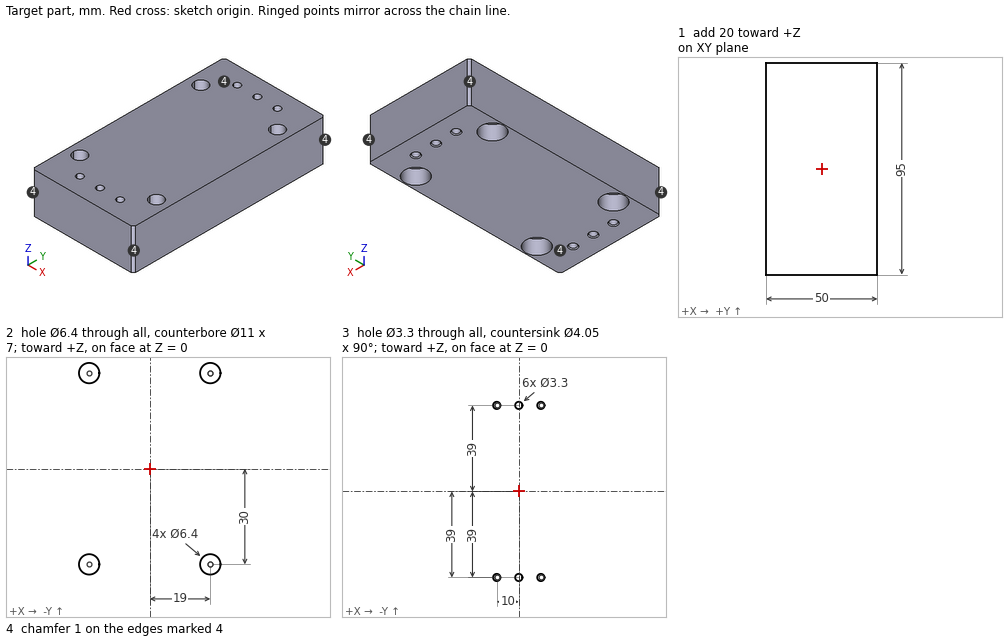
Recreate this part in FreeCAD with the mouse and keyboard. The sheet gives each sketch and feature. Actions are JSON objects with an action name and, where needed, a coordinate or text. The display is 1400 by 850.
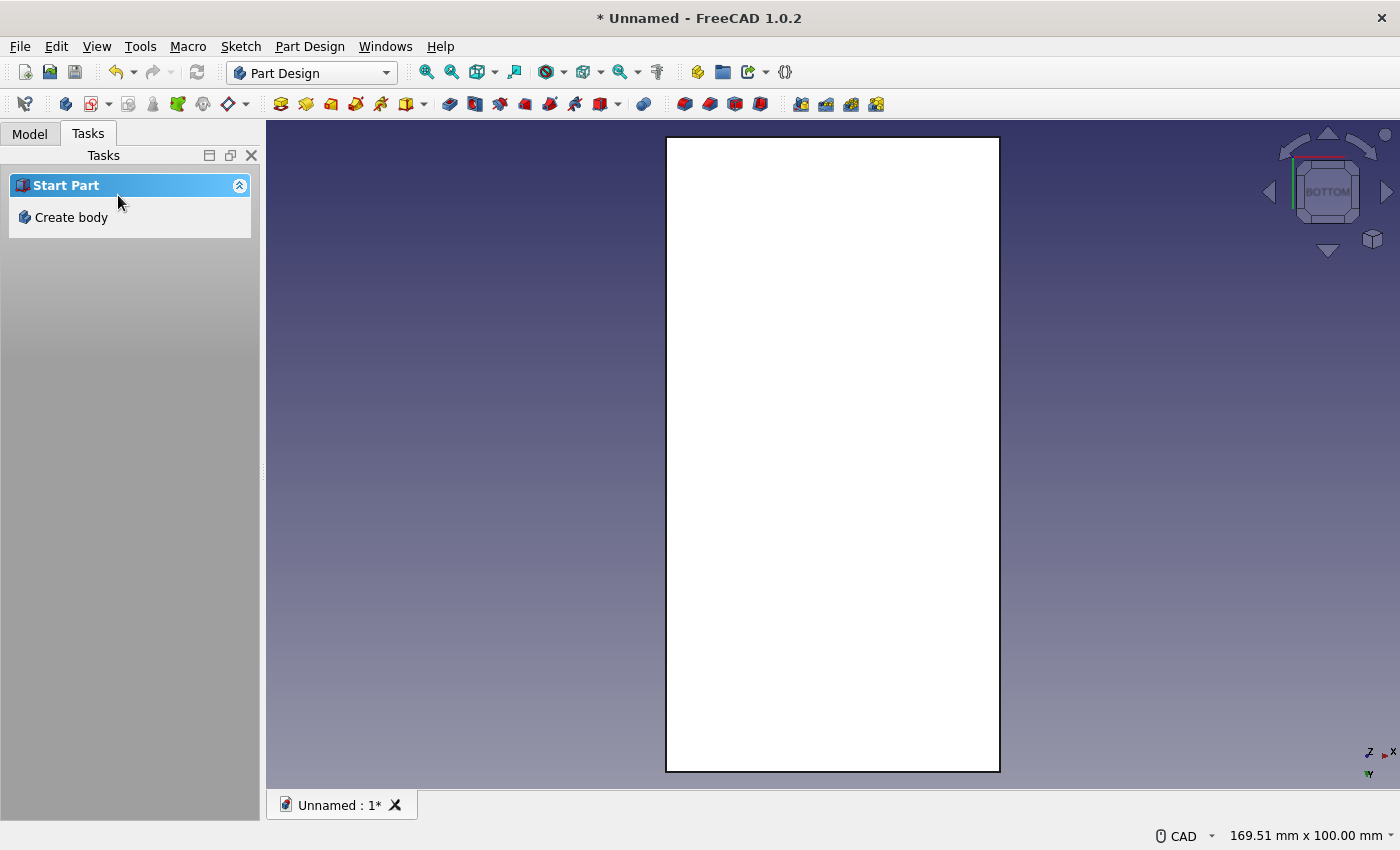
{"action": "left_click", "coordinate": [833, 544]}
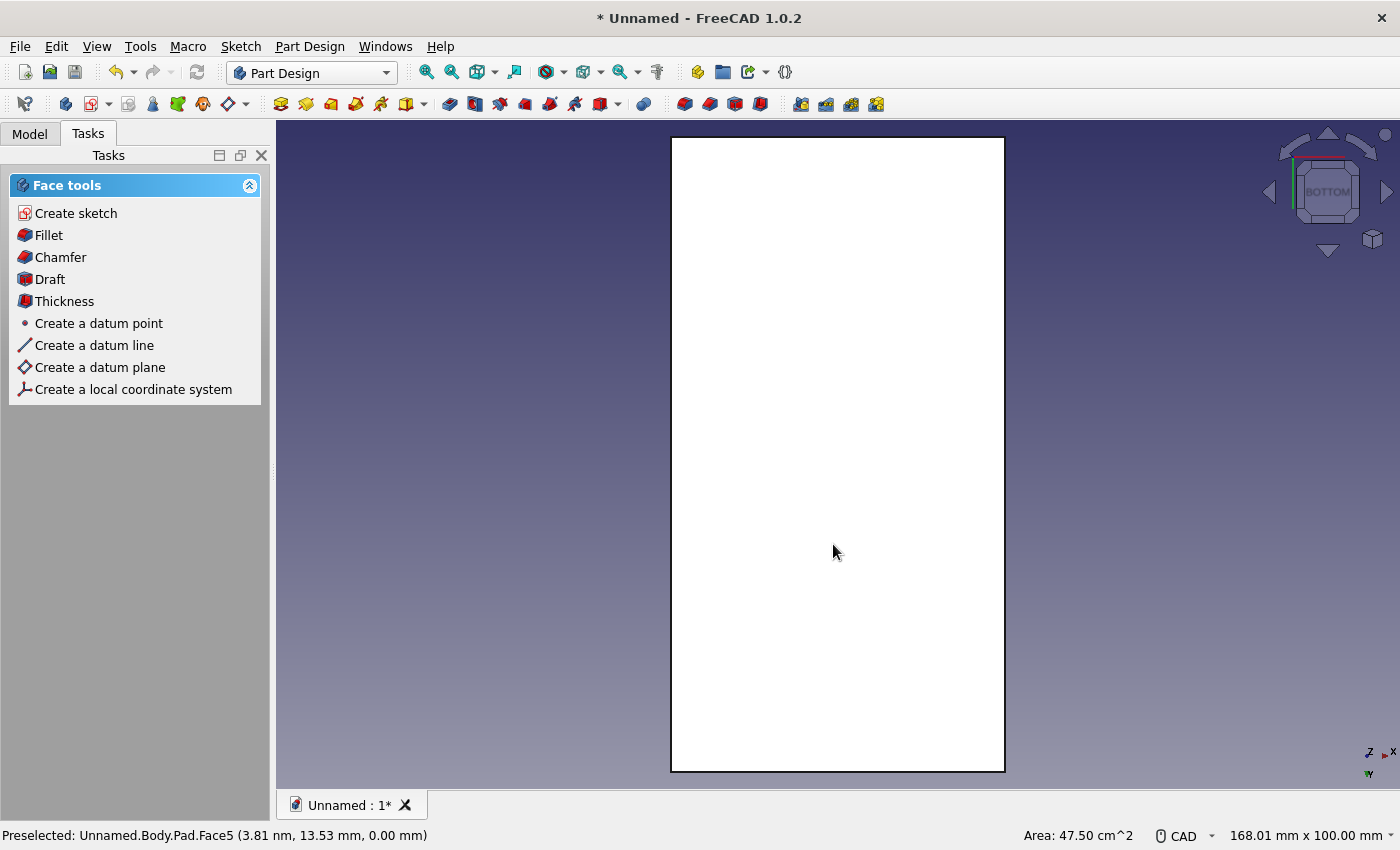
{"action": "left_click", "coordinate": [90, 104]}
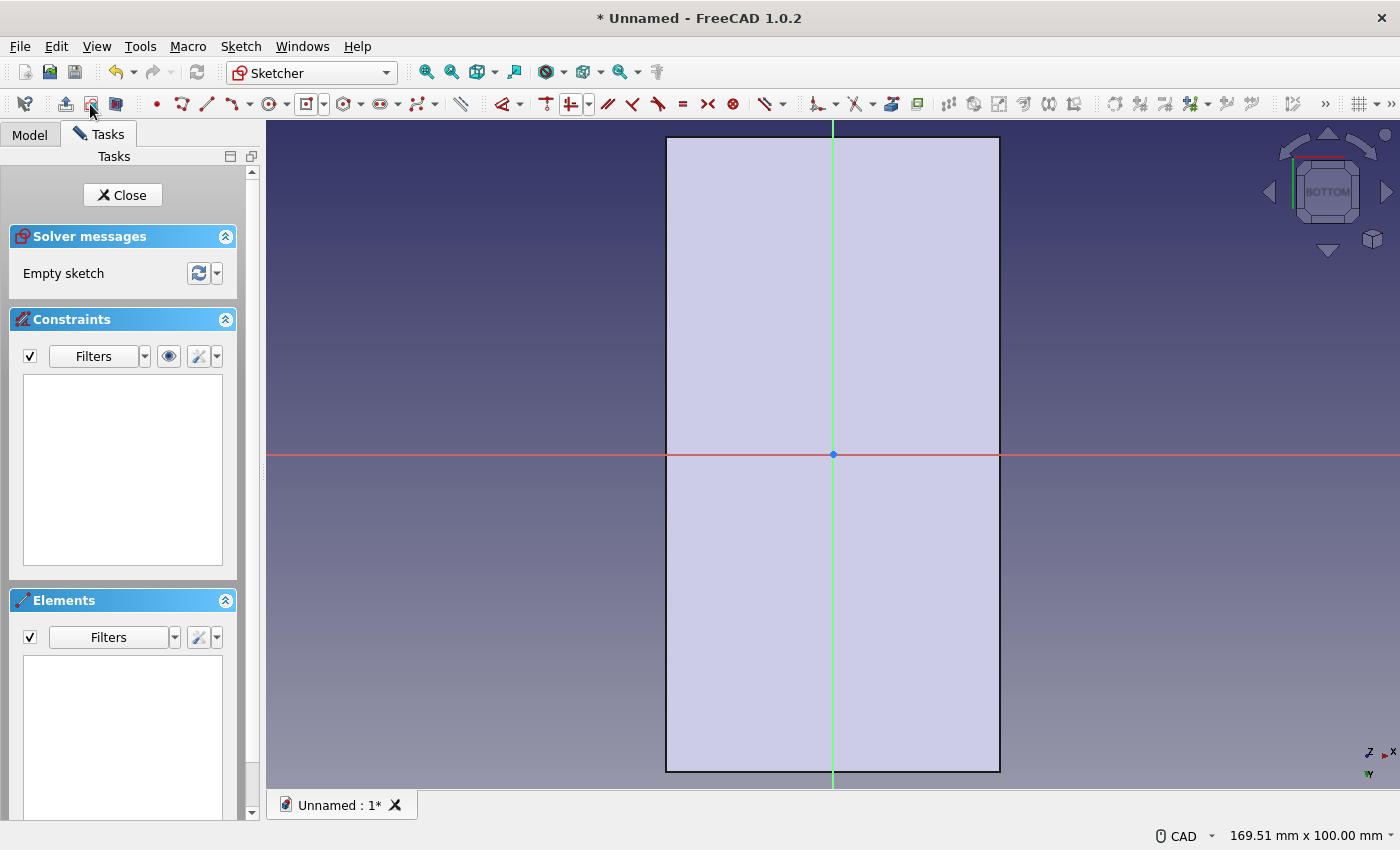
{"action": "left_click", "coordinate": [268, 104]}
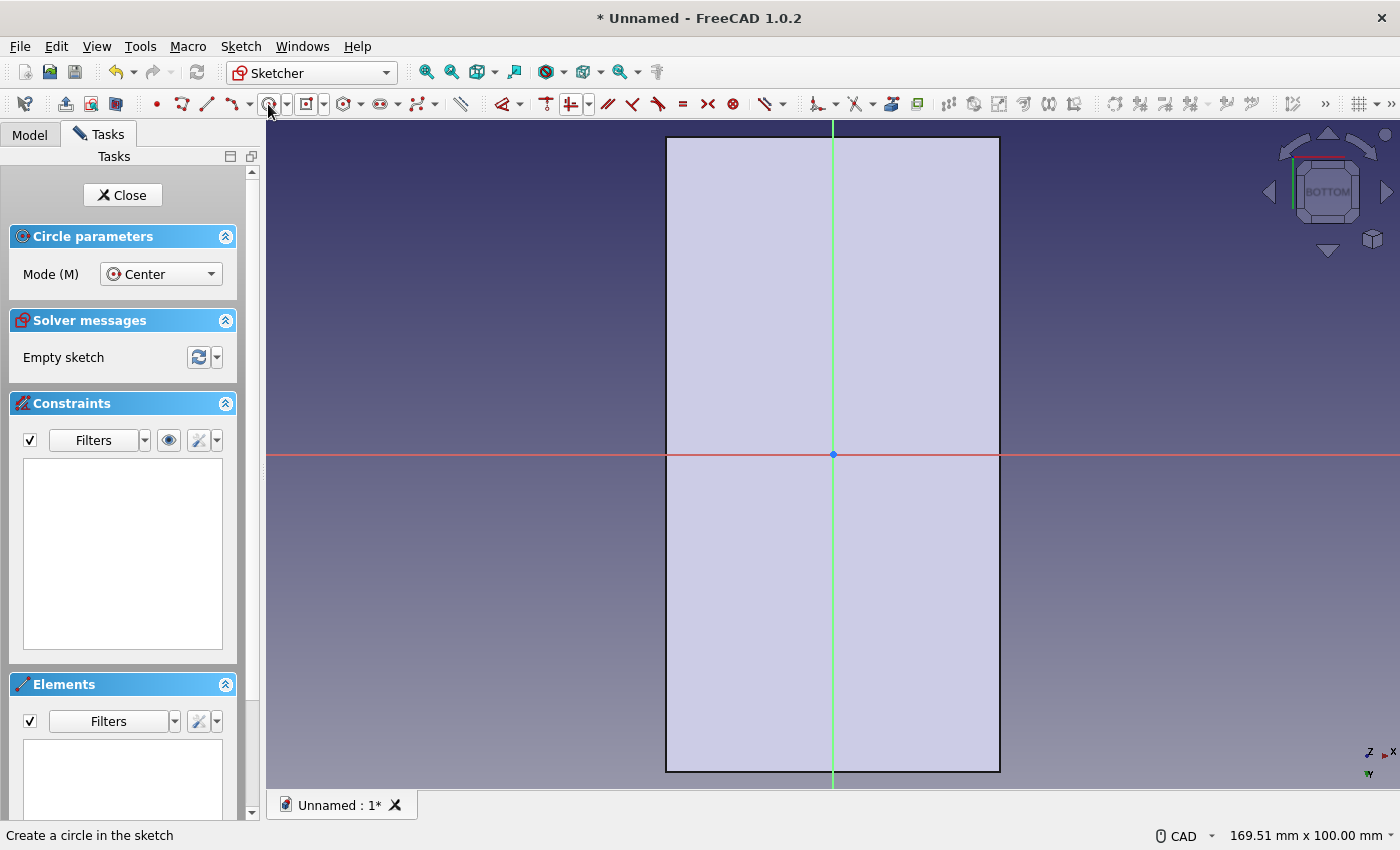
{"action": "left_click", "coordinate": [960, 655]}
{"action": "left_click", "coordinate": [975, 640]}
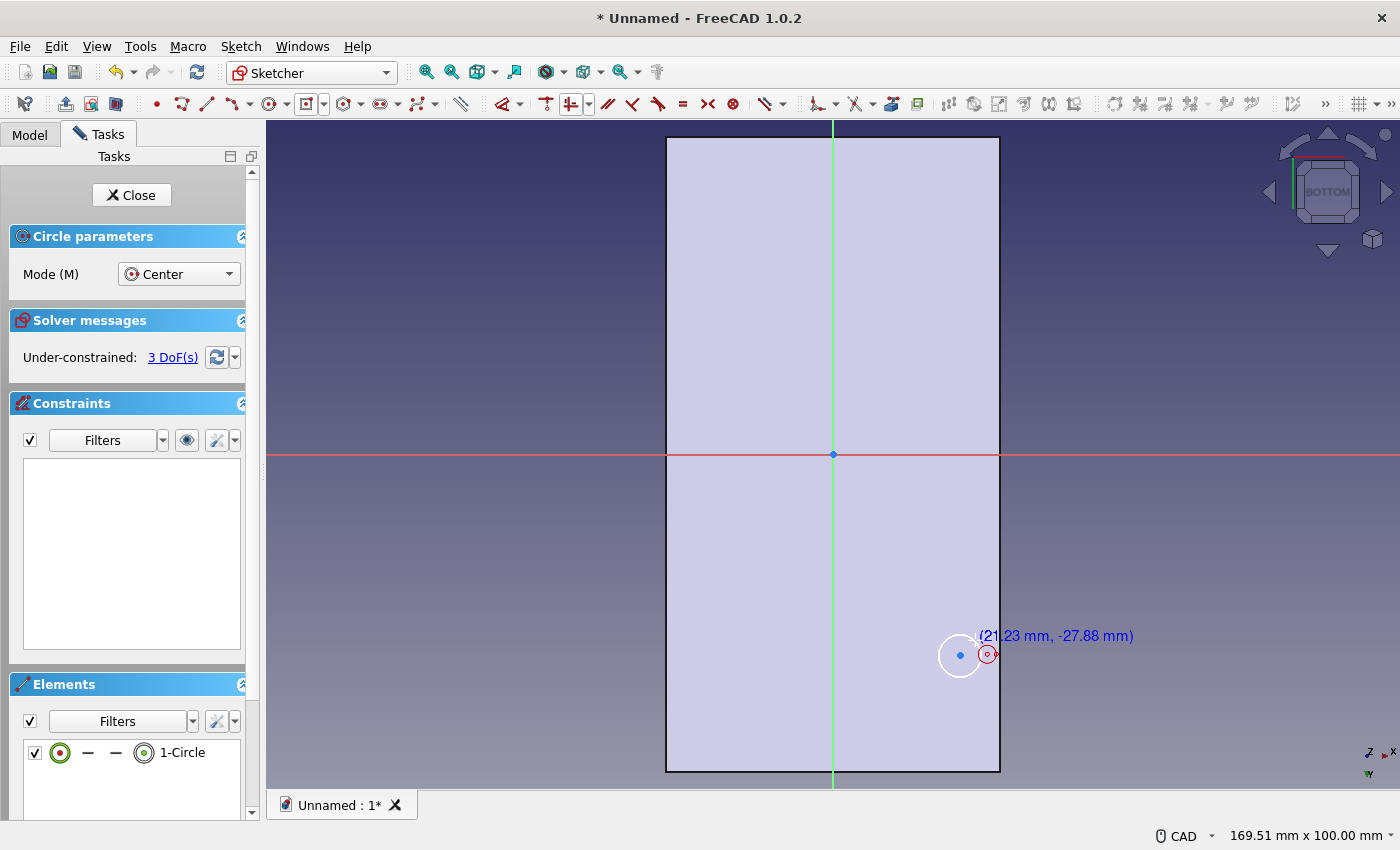
{"action": "left_click", "coordinate": [960, 254]}
{"action": "left_click", "coordinate": [975, 239]}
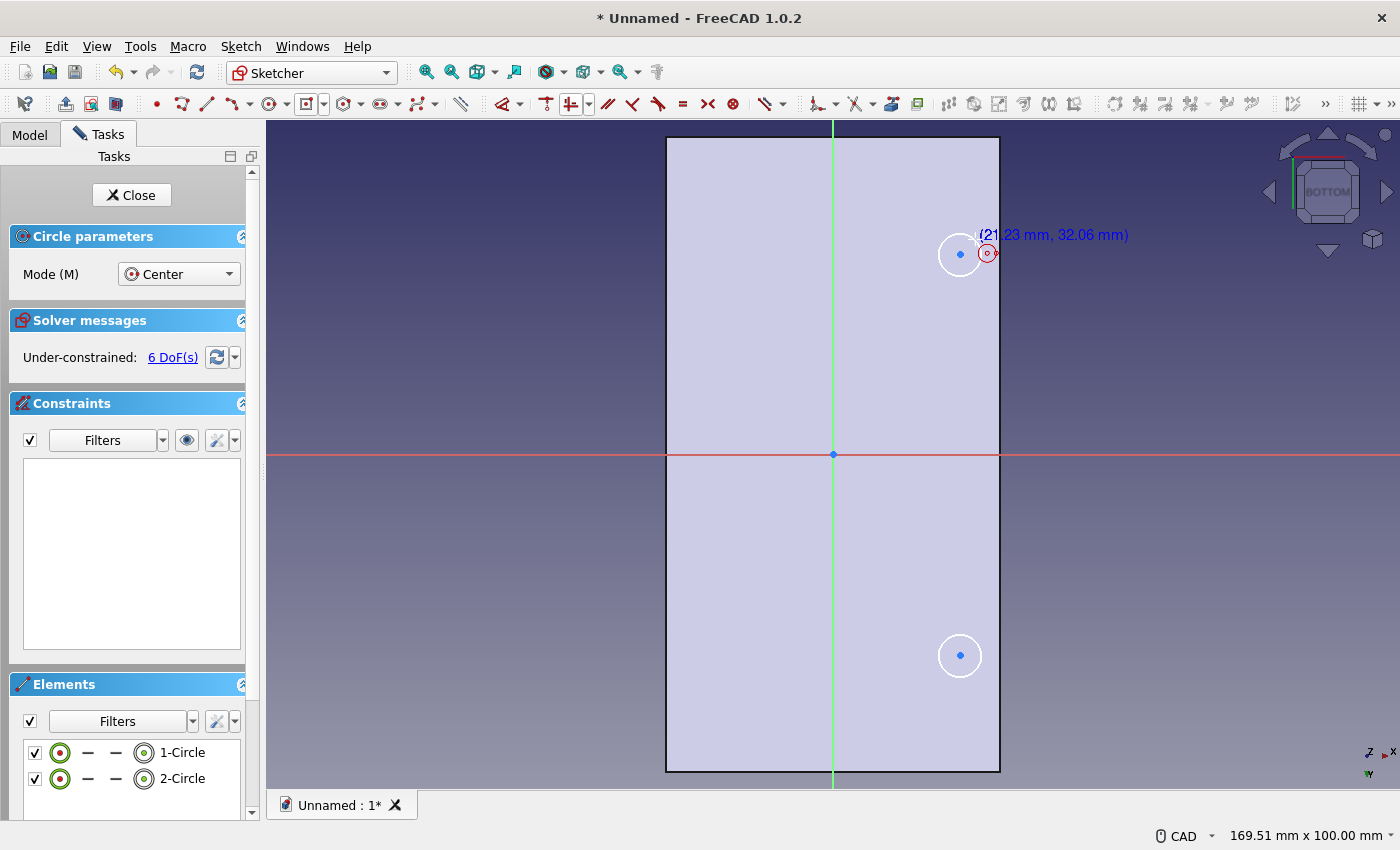
{"action": "left_click", "coordinate": [706, 254]}
{"action": "left_click", "coordinate": [721, 239]}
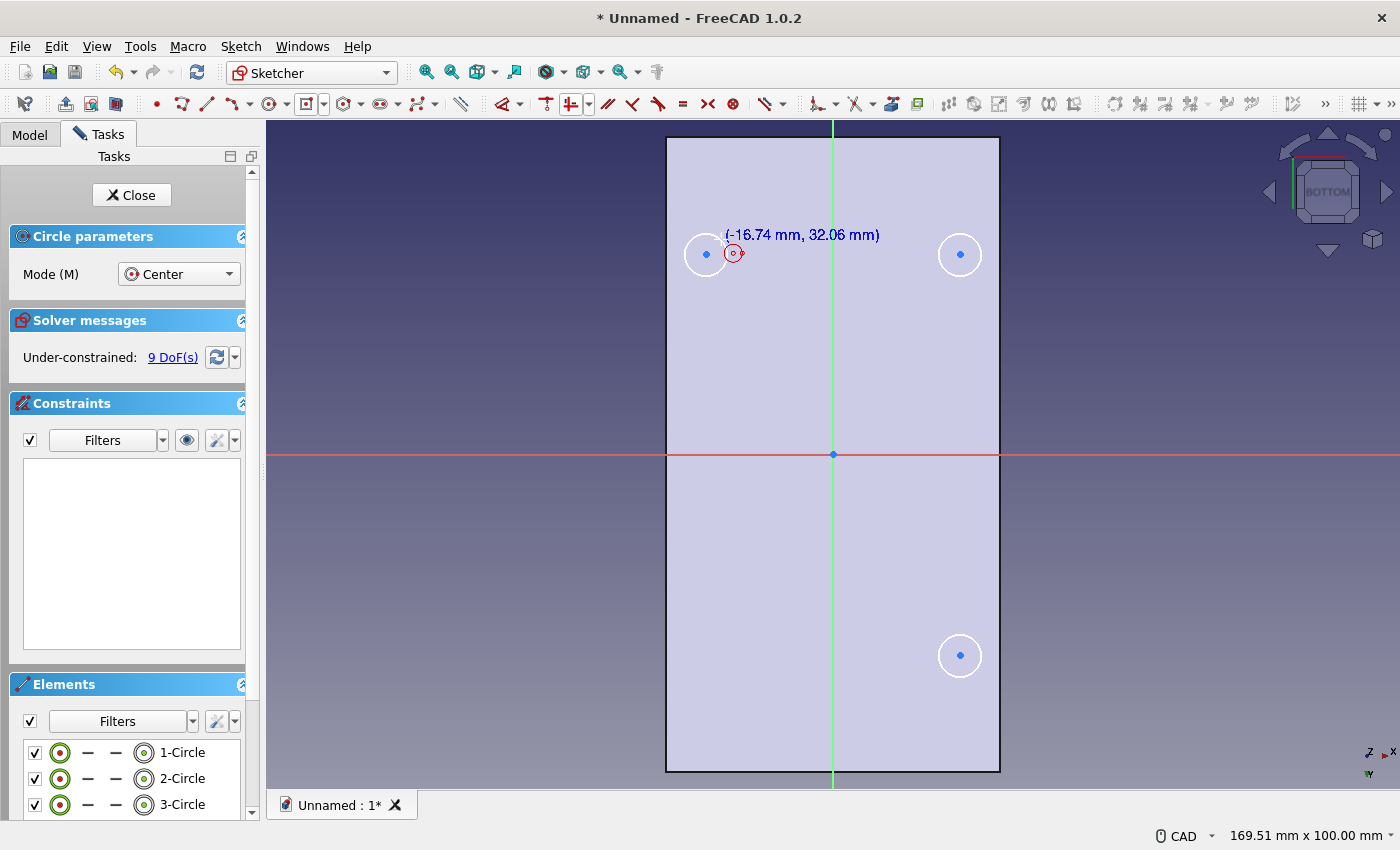
{"action": "left_click", "coordinate": [706, 655]}
{"action": "left_click", "coordinate": [721, 640]}
{"action": "key", "text": "Escape"}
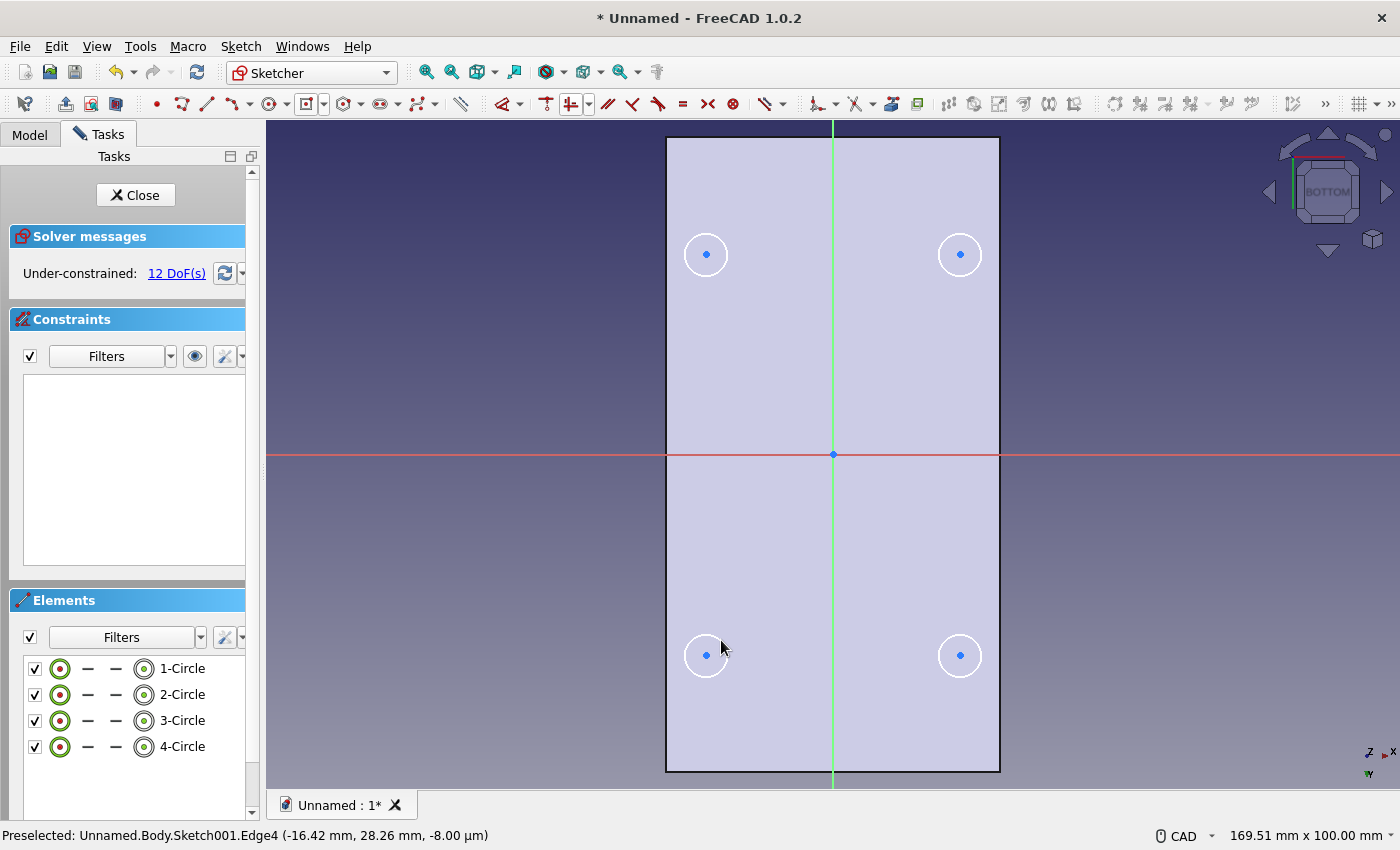
{"action": "left_click", "coordinate": [975, 641]}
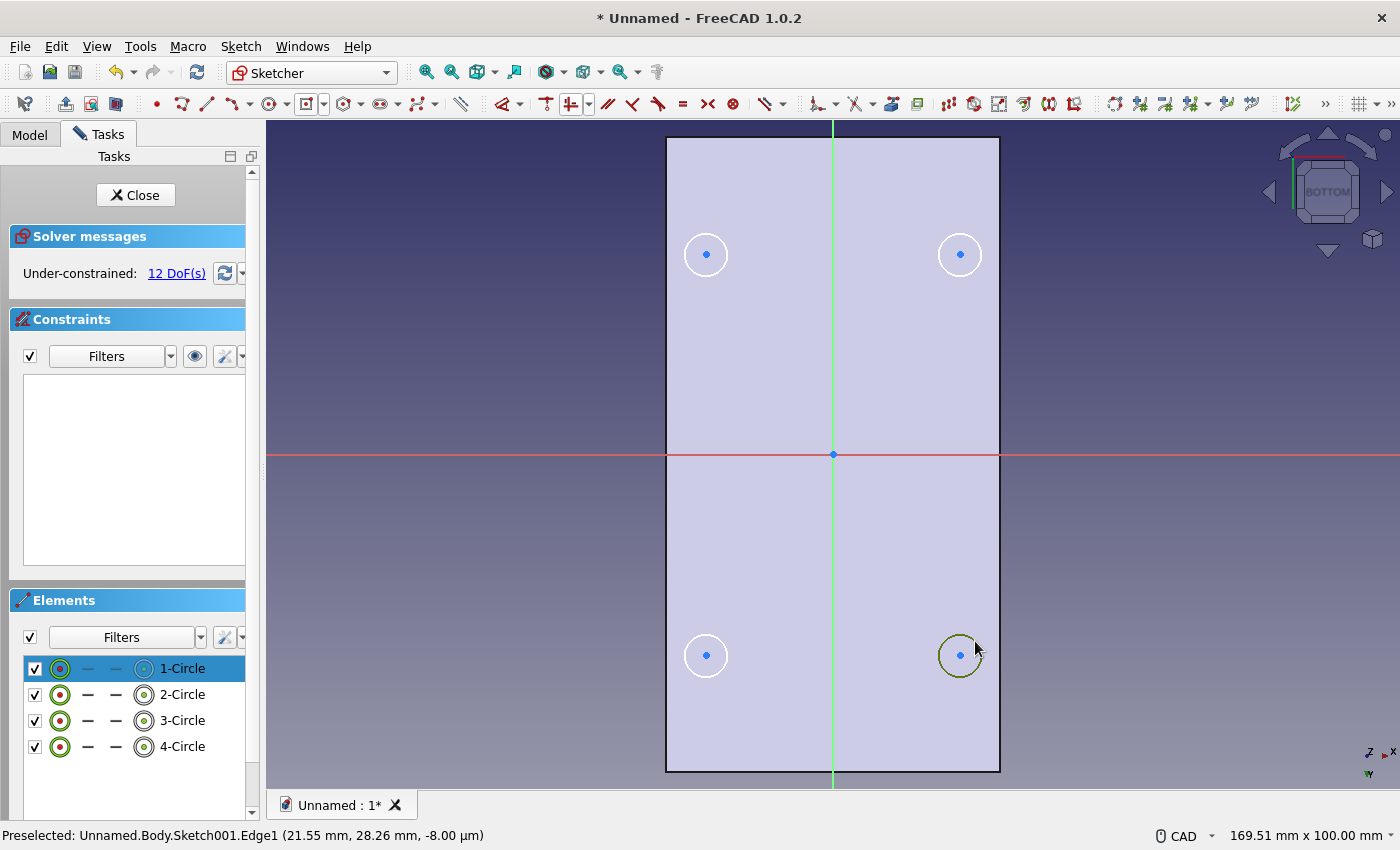
{"action": "left_click", "coordinate": [975, 240]}